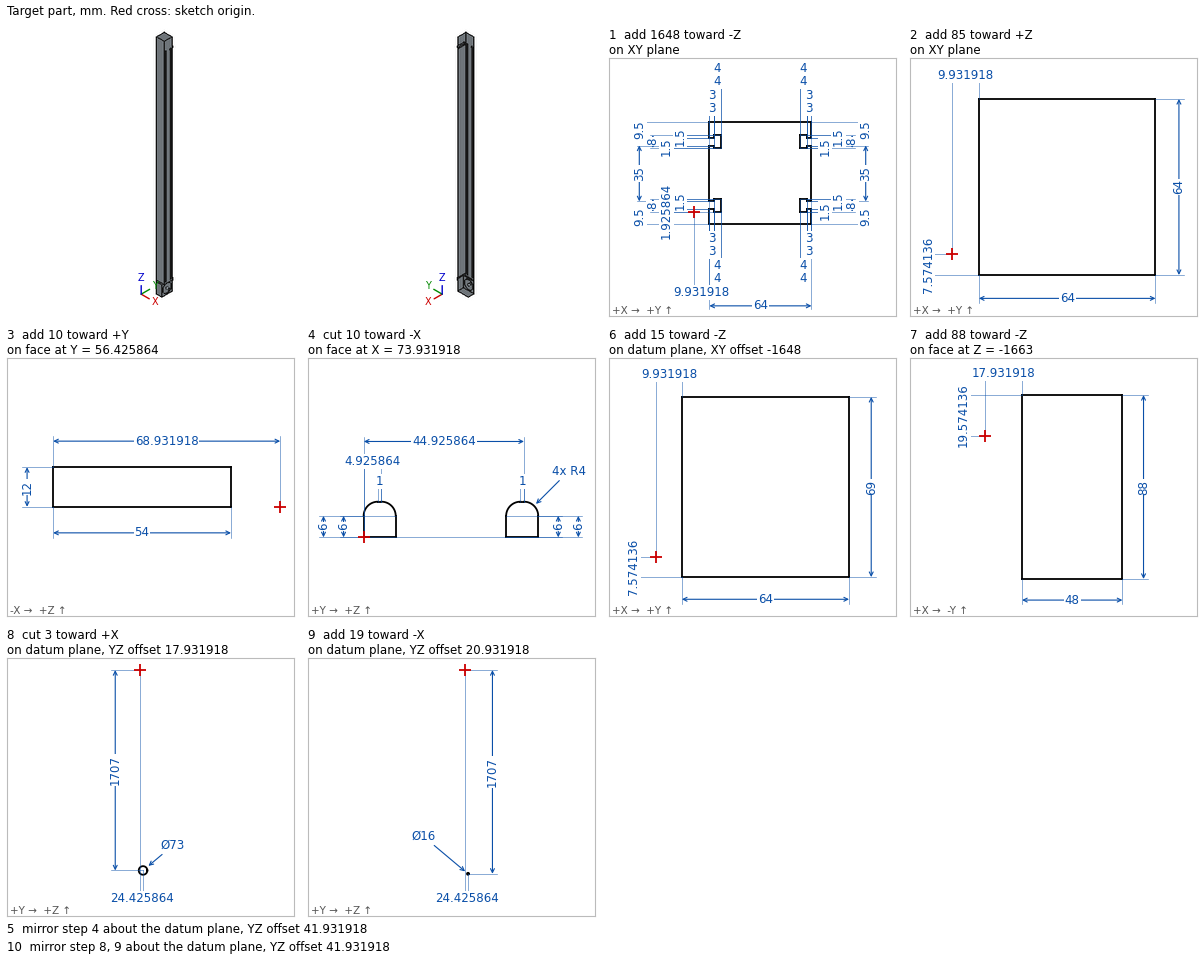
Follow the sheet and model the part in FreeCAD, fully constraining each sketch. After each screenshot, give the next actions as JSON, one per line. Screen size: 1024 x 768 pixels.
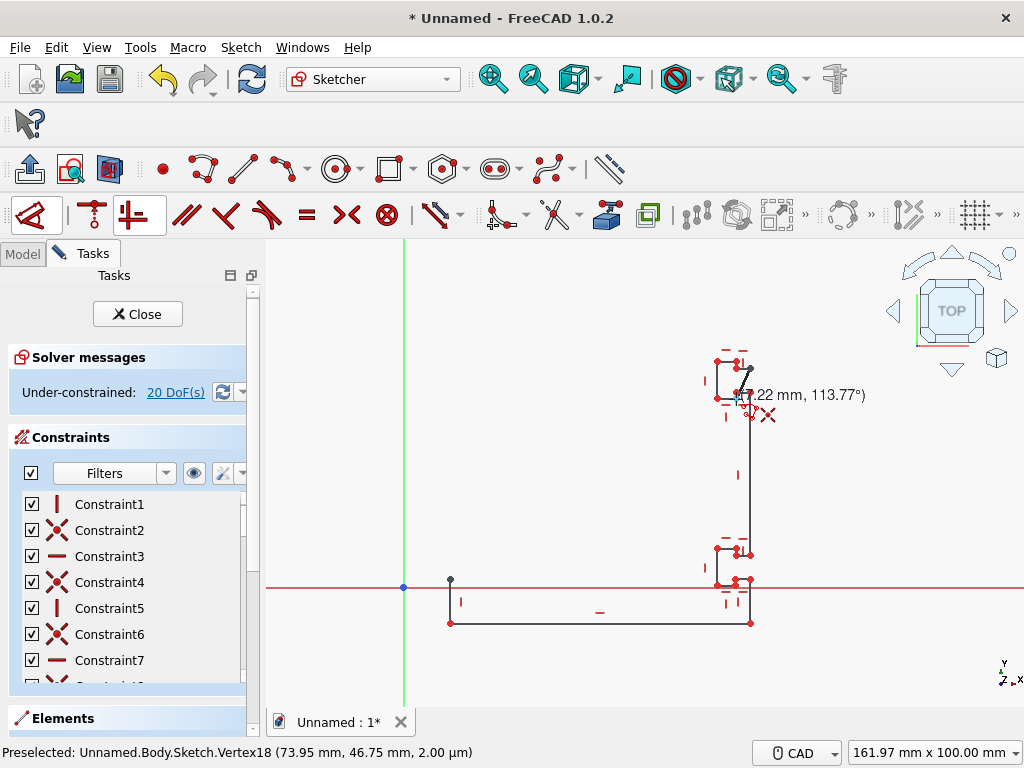
{"action": "left_click", "coordinate": [750, 324]}
{"action": "left_click", "coordinate": [450, 324]}
{"action": "left_click", "coordinate": [450, 368]}
{"action": "left_click", "coordinate": [464, 368]}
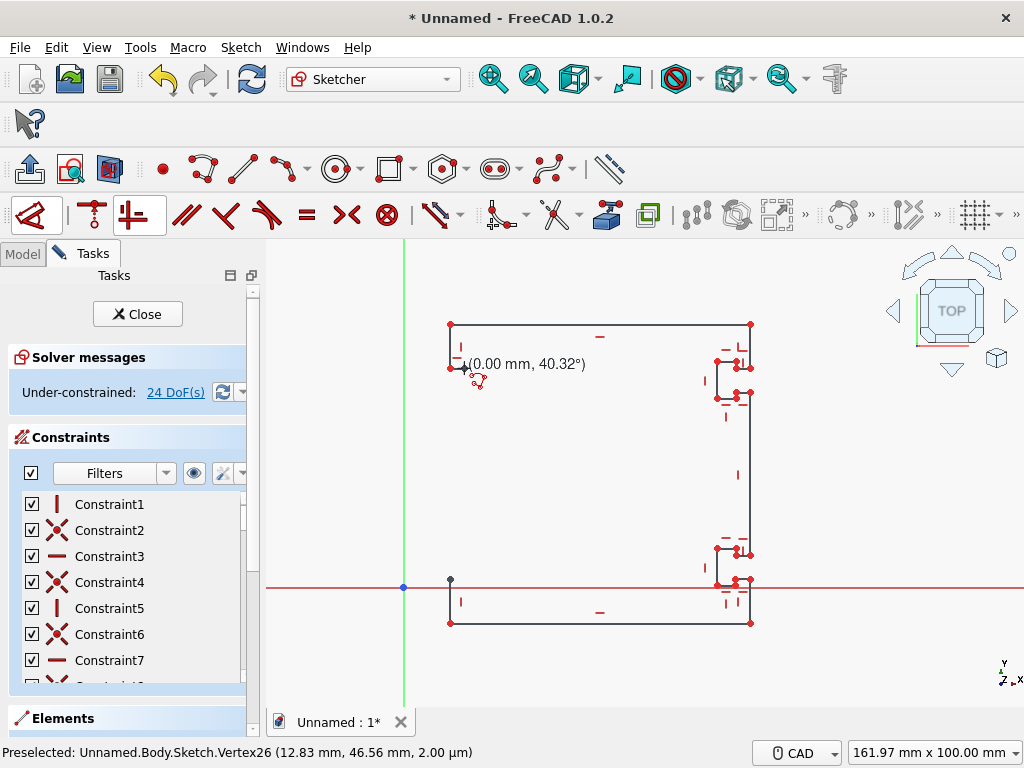
{"action": "scroll", "coordinate": [464, 361], "scroll_direction": "up", "scroll_amount": 5}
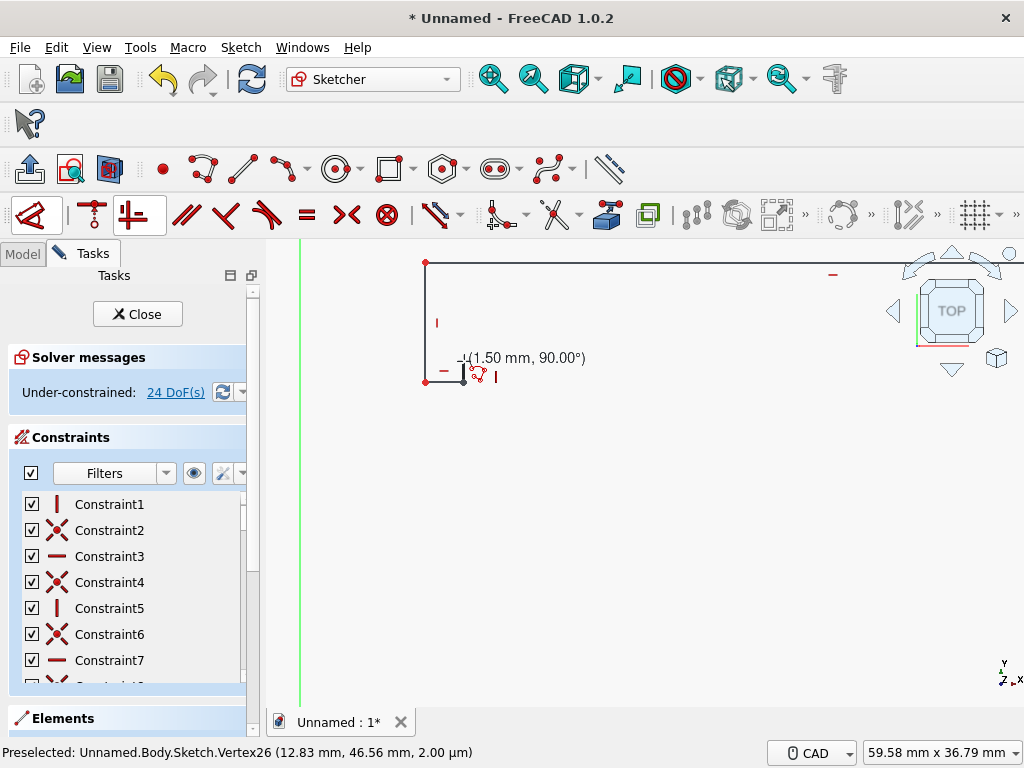
{"action": "left_click", "coordinate": [464, 361]}
{"action": "left_click", "coordinate": [516, 361]}
{"action": "left_click", "coordinate": [516, 463]}
{"action": "left_click", "coordinate": [465, 463]}
{"action": "left_click", "coordinate": [465, 444]}
{"action": "left_click", "coordinate": [427, 444]}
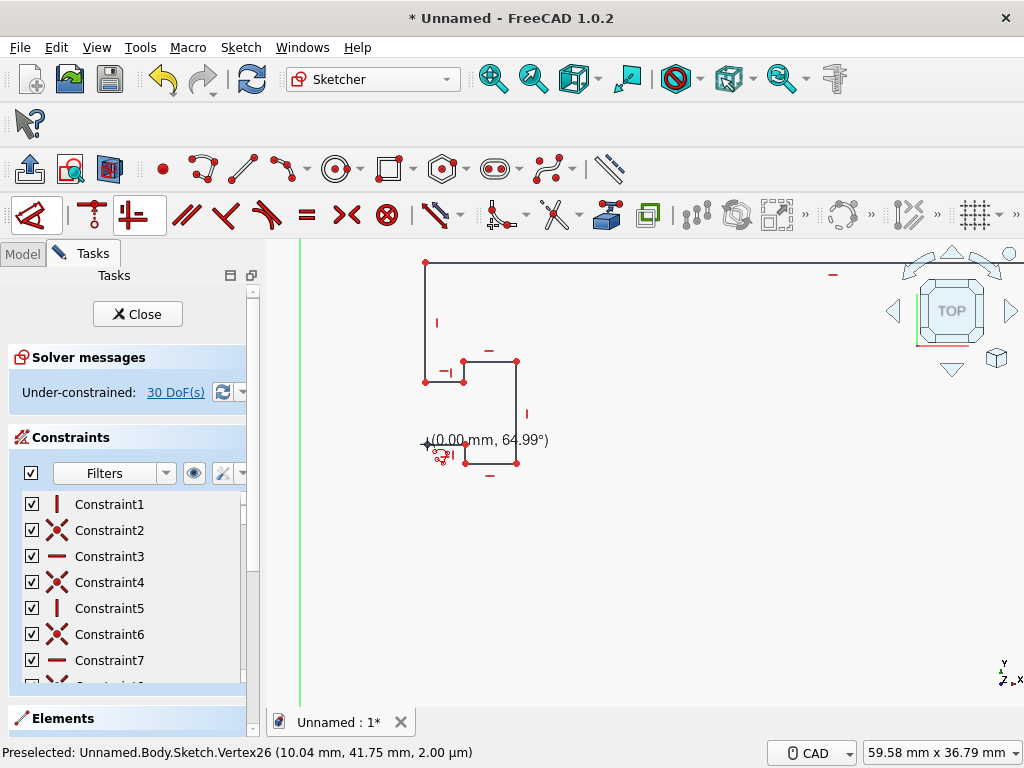
{"action": "scroll", "coordinate": [464, 360], "scroll_direction": "down", "scroll_amount": 5}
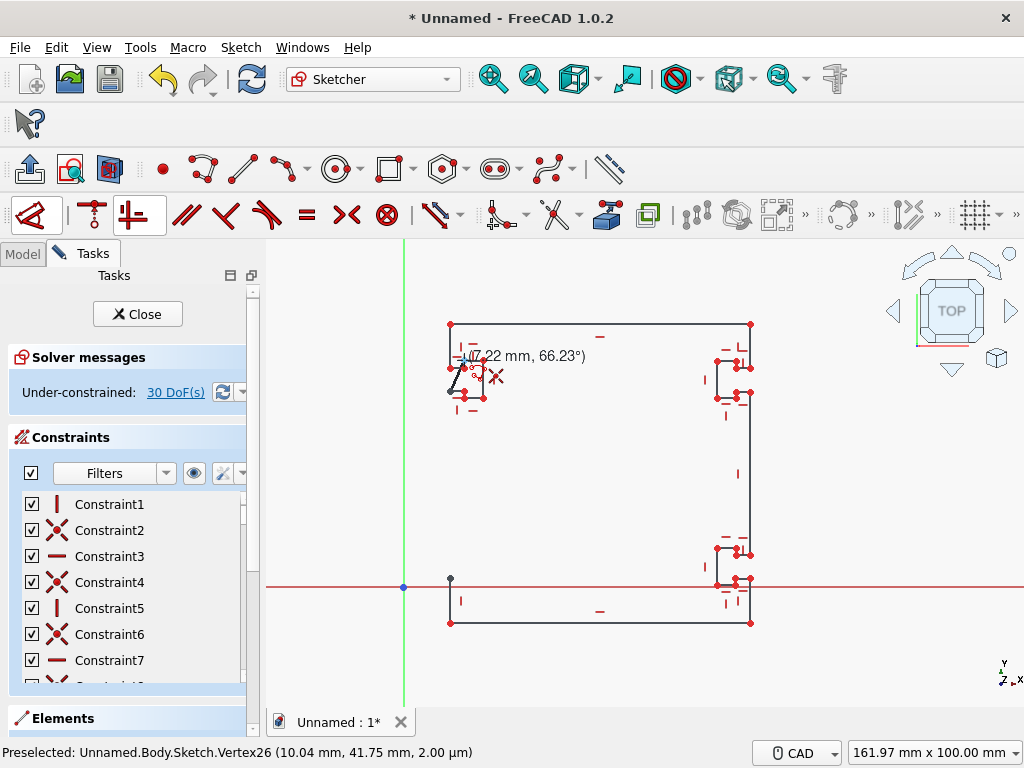
{"action": "left_click", "coordinate": [451, 555]}
{"action": "left_click", "coordinate": [464, 555]}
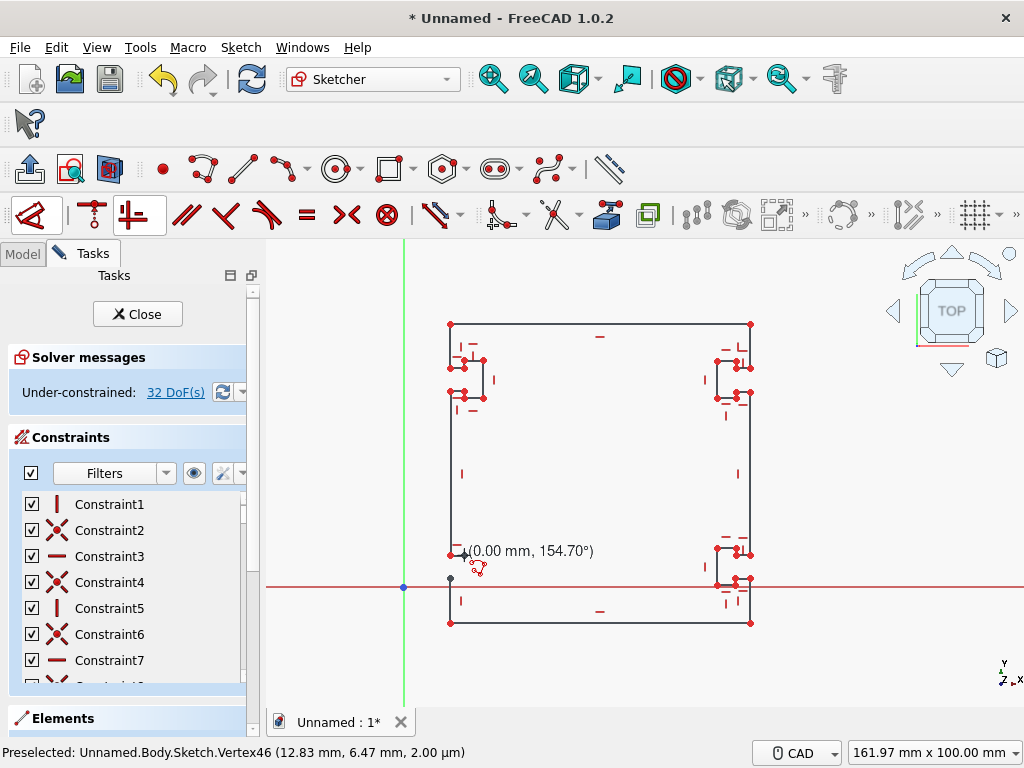
{"action": "scroll", "coordinate": [464, 548], "scroll_direction": "up", "scroll_amount": 5}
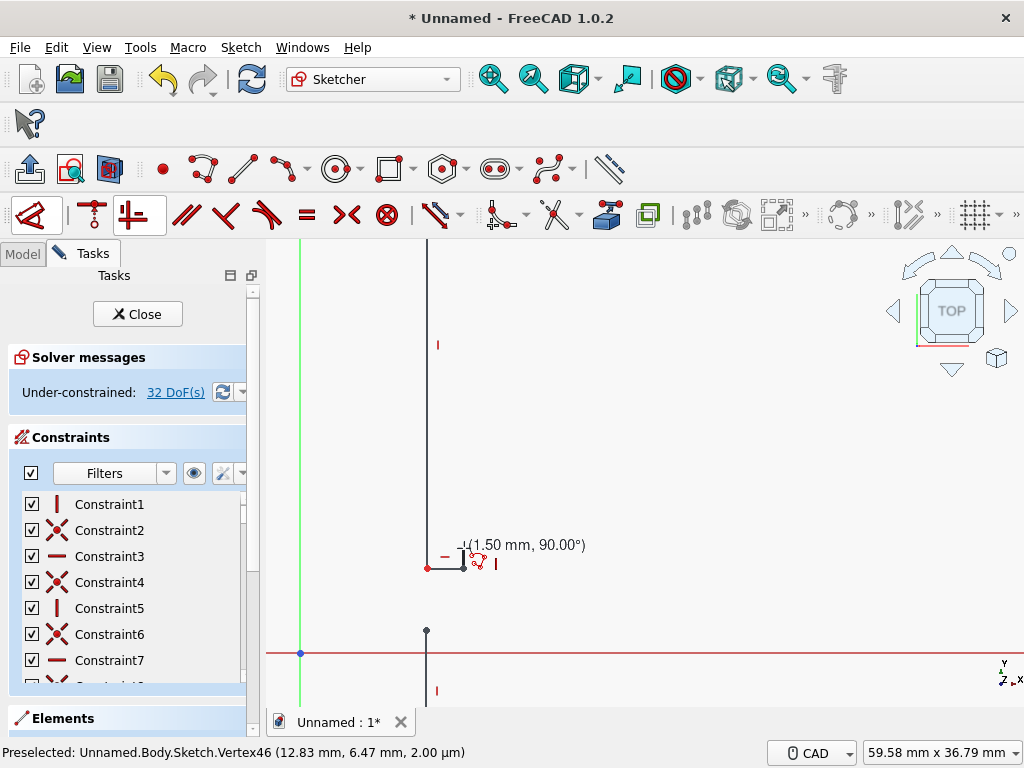
{"action": "left_click", "coordinate": [464, 546]}
{"action": "left_click", "coordinate": [516, 546]}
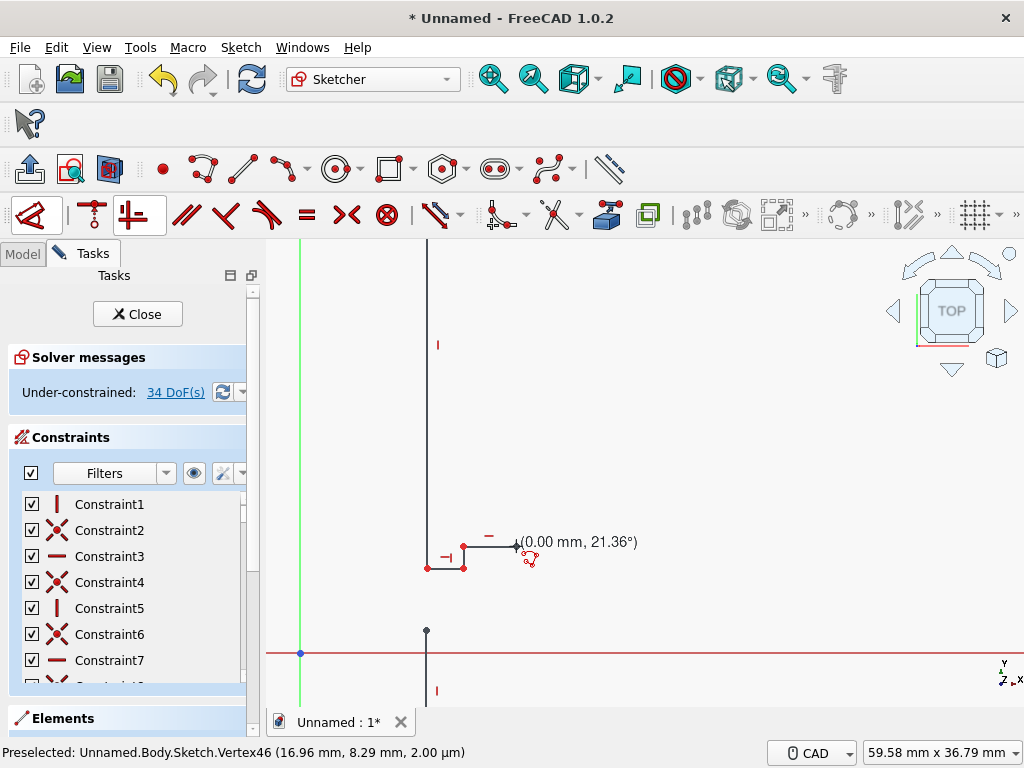
{"action": "scroll", "coordinate": [516, 648], "scroll_direction": "up", "scroll_amount": 6}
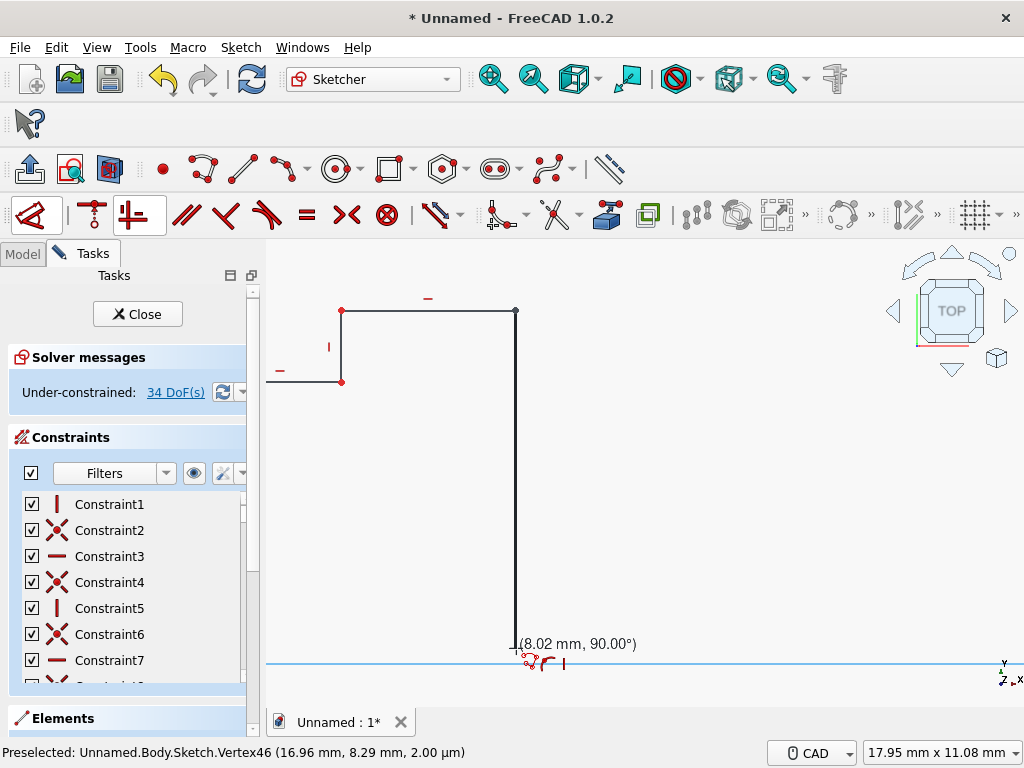
{"action": "left_click", "coordinate": [515, 646]}
{"action": "left_click", "coordinate": [345, 646]}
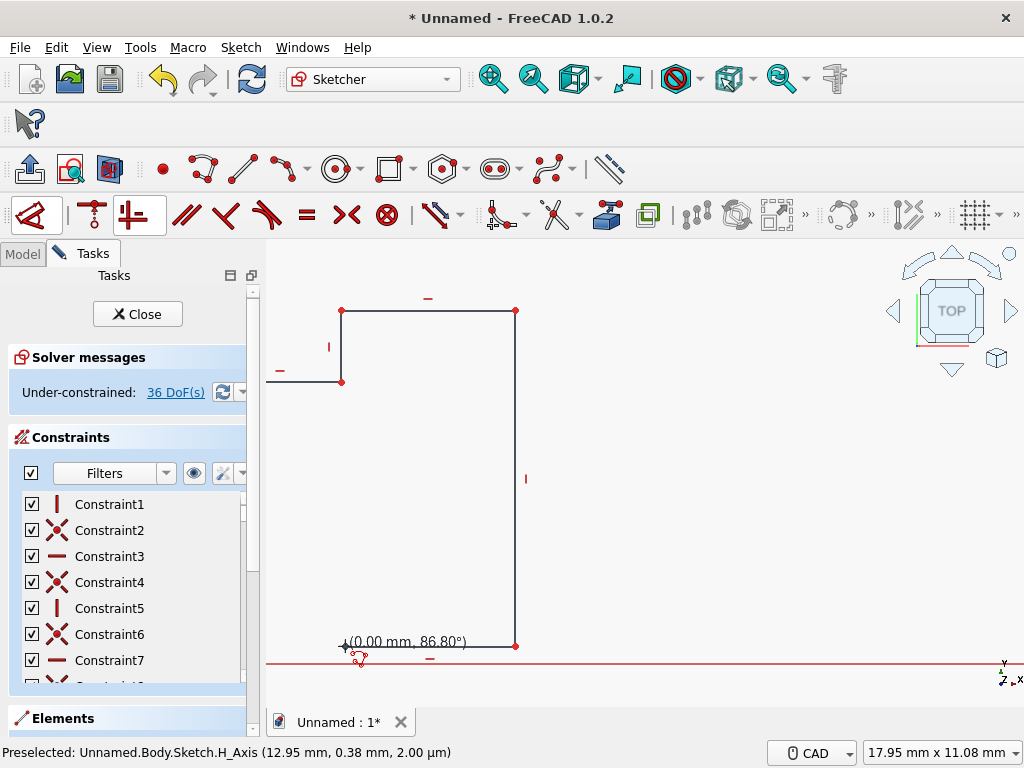
{"action": "scroll", "coordinate": [479, 578], "scroll_direction": "down", "scroll_amount": 11}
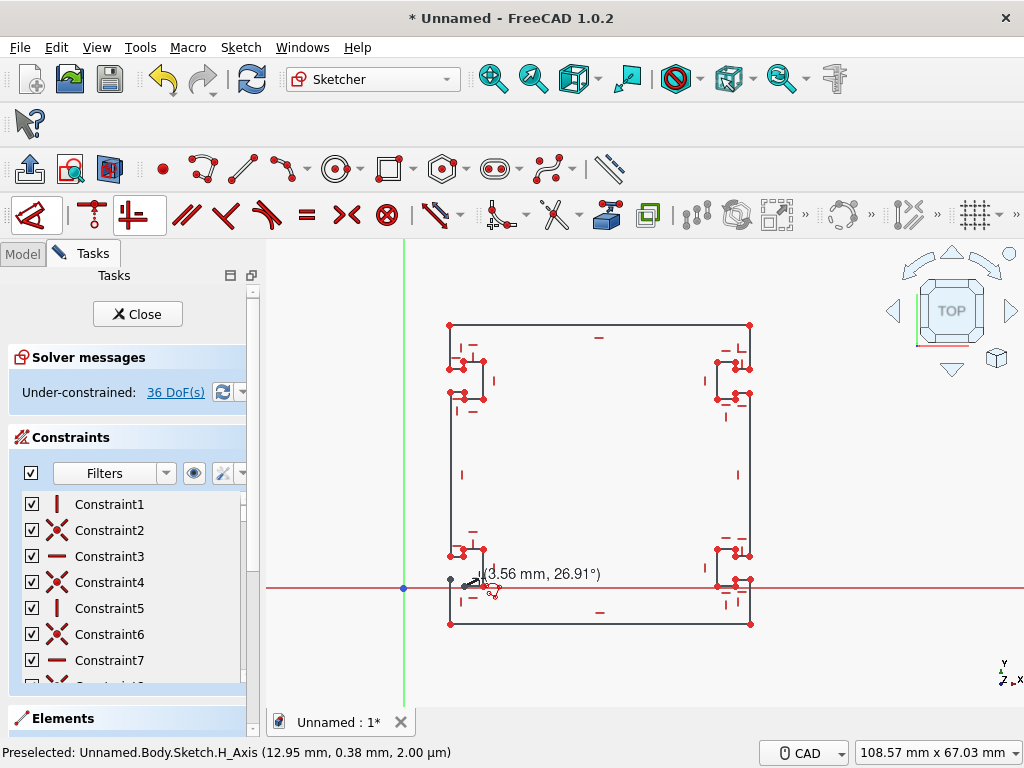
{"action": "scroll", "coordinate": [464, 579], "scroll_direction": "up", "scroll_amount": 5}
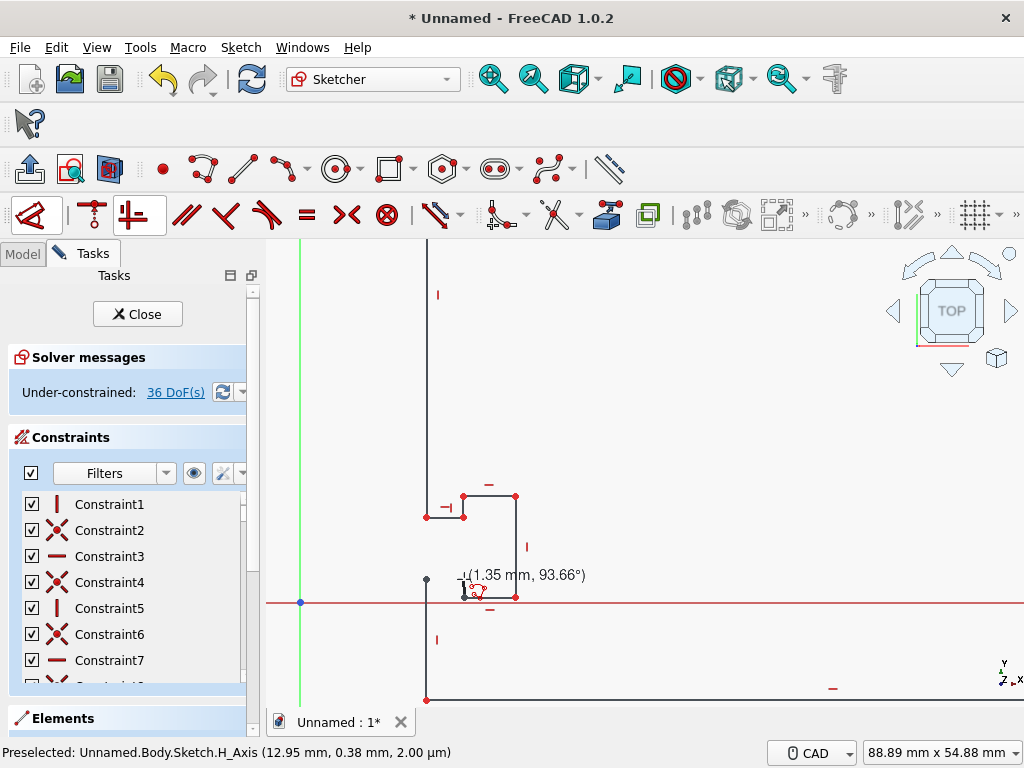
{"action": "left_click", "coordinate": [465, 578]}
{"action": "left_click", "coordinate": [426, 580]}
{"action": "key", "text": "Escape"}
{"action": "key", "text": "Escape"}